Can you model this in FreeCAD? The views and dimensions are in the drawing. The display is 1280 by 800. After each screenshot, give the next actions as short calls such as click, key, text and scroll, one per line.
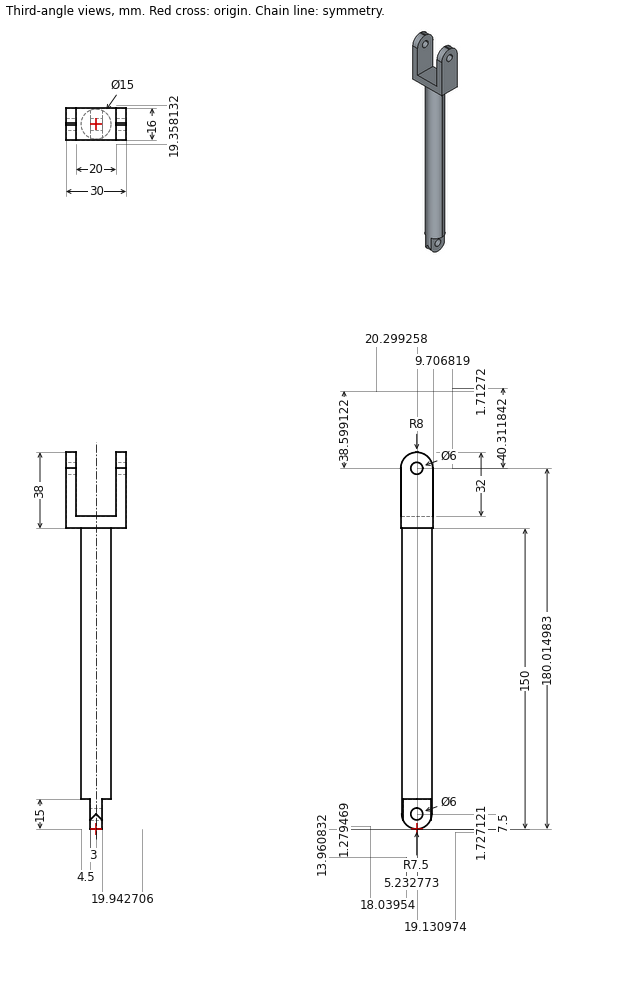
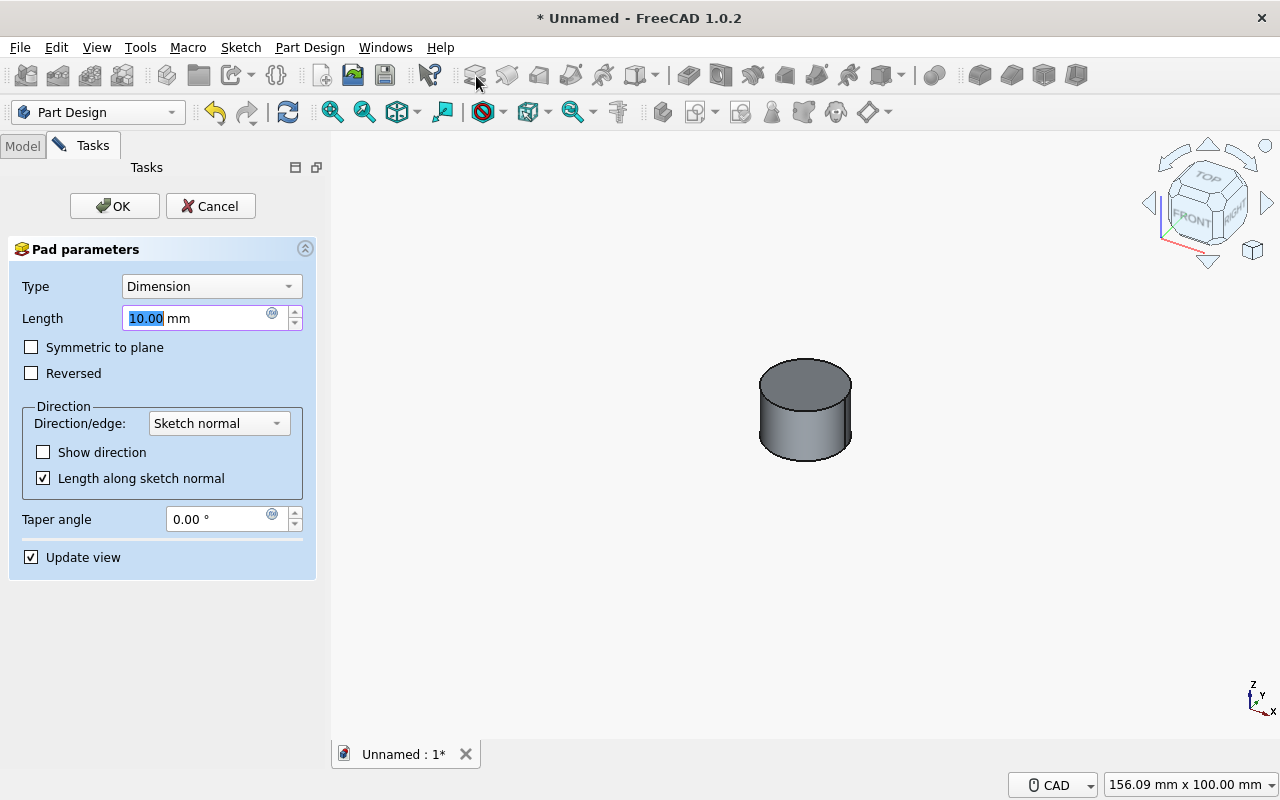
text(150)
key(Tab)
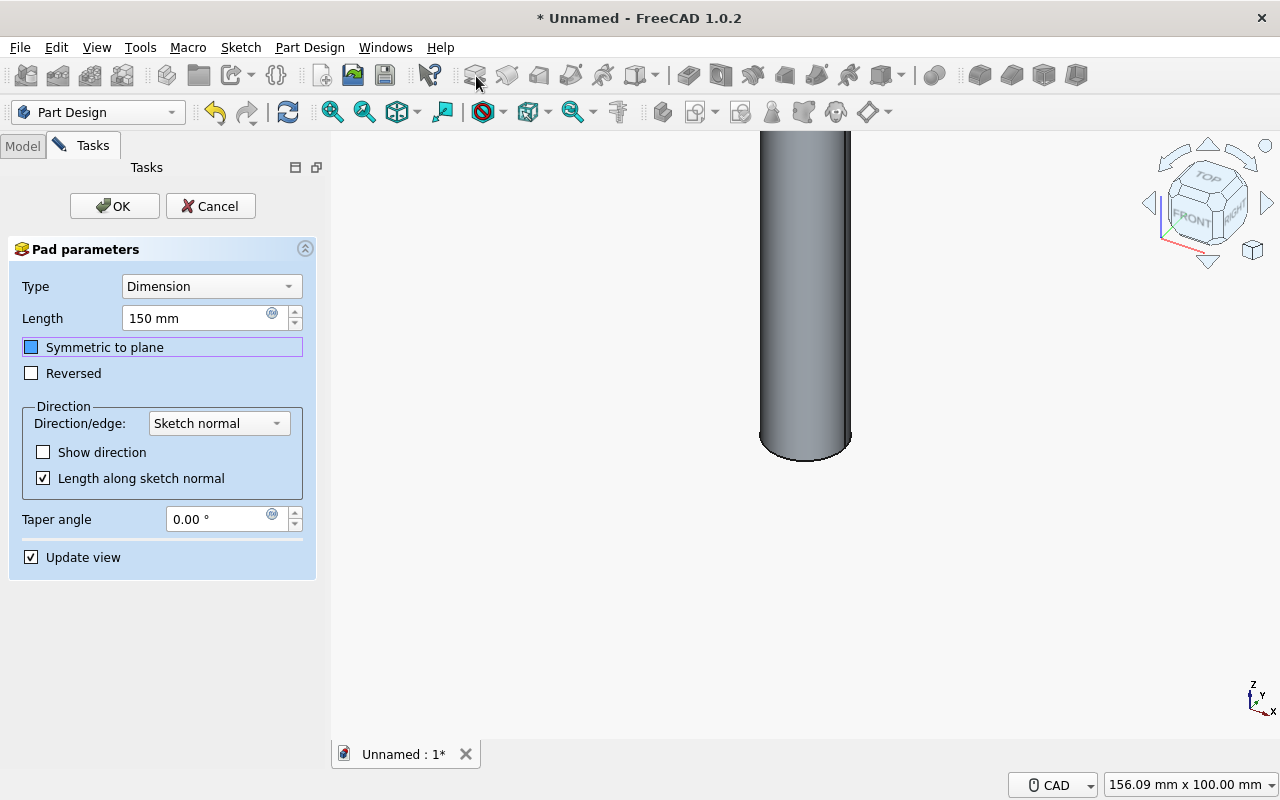
click(115, 206)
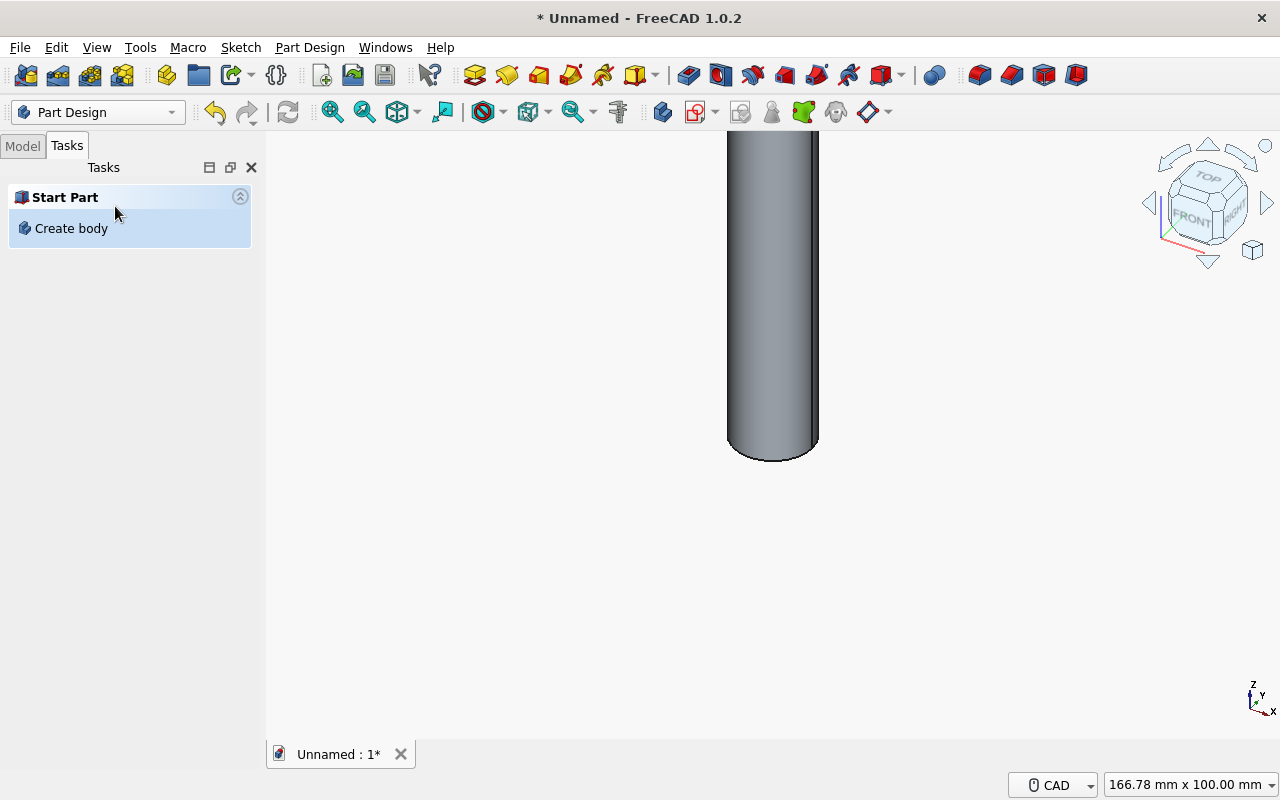
key(v)
key(f)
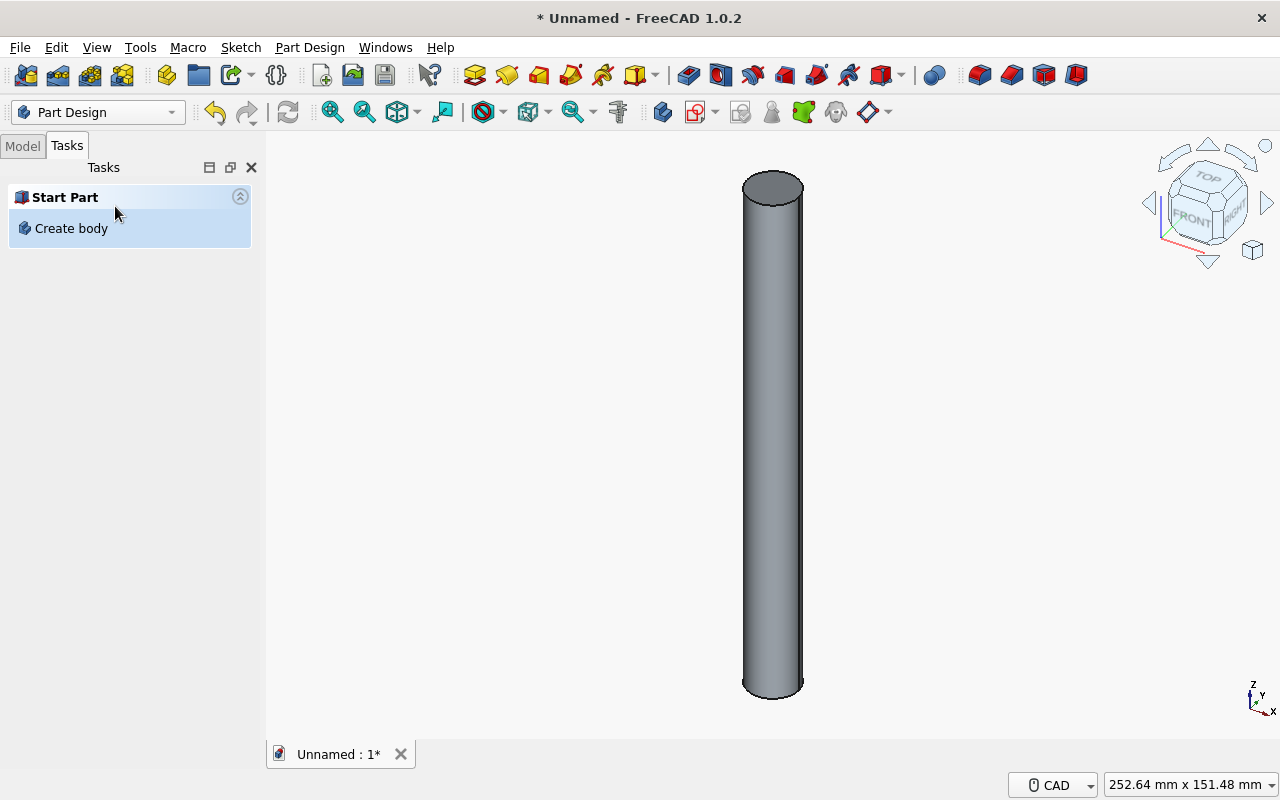
click(773, 187)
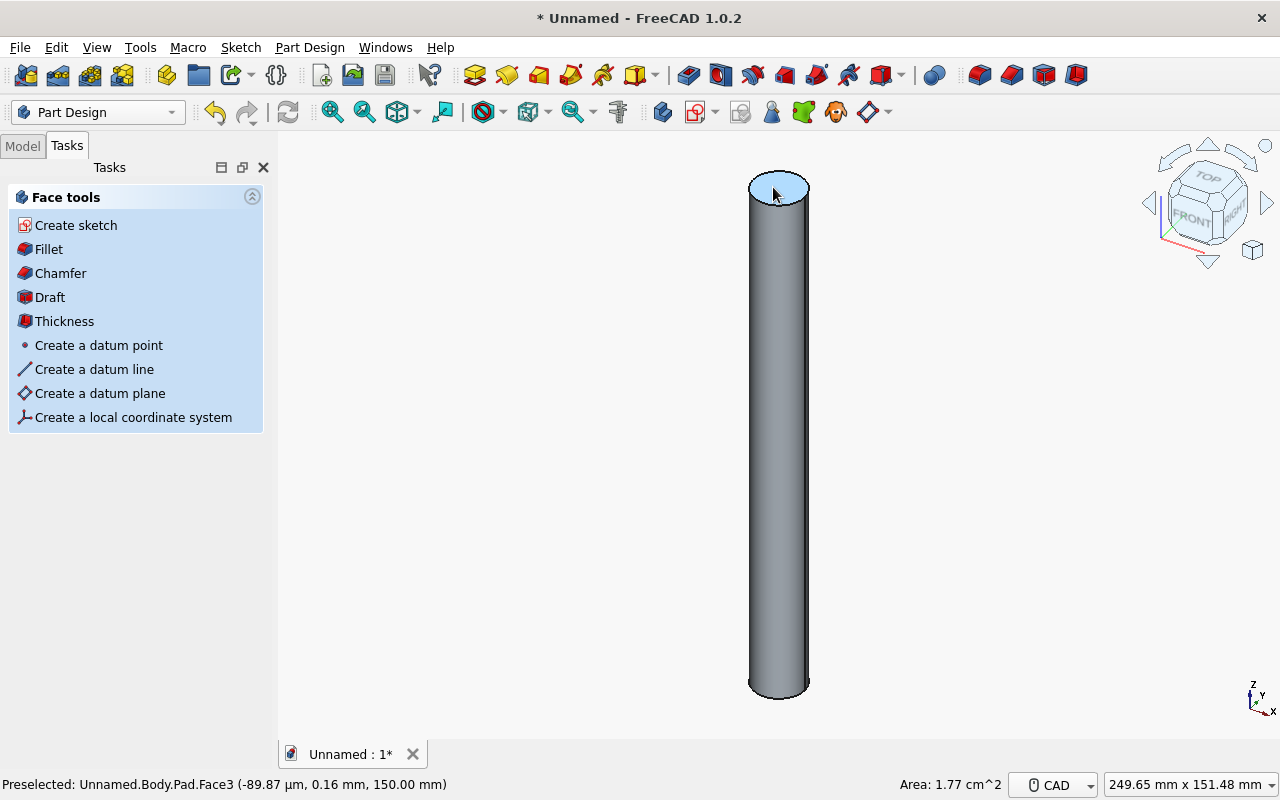
click(696, 112)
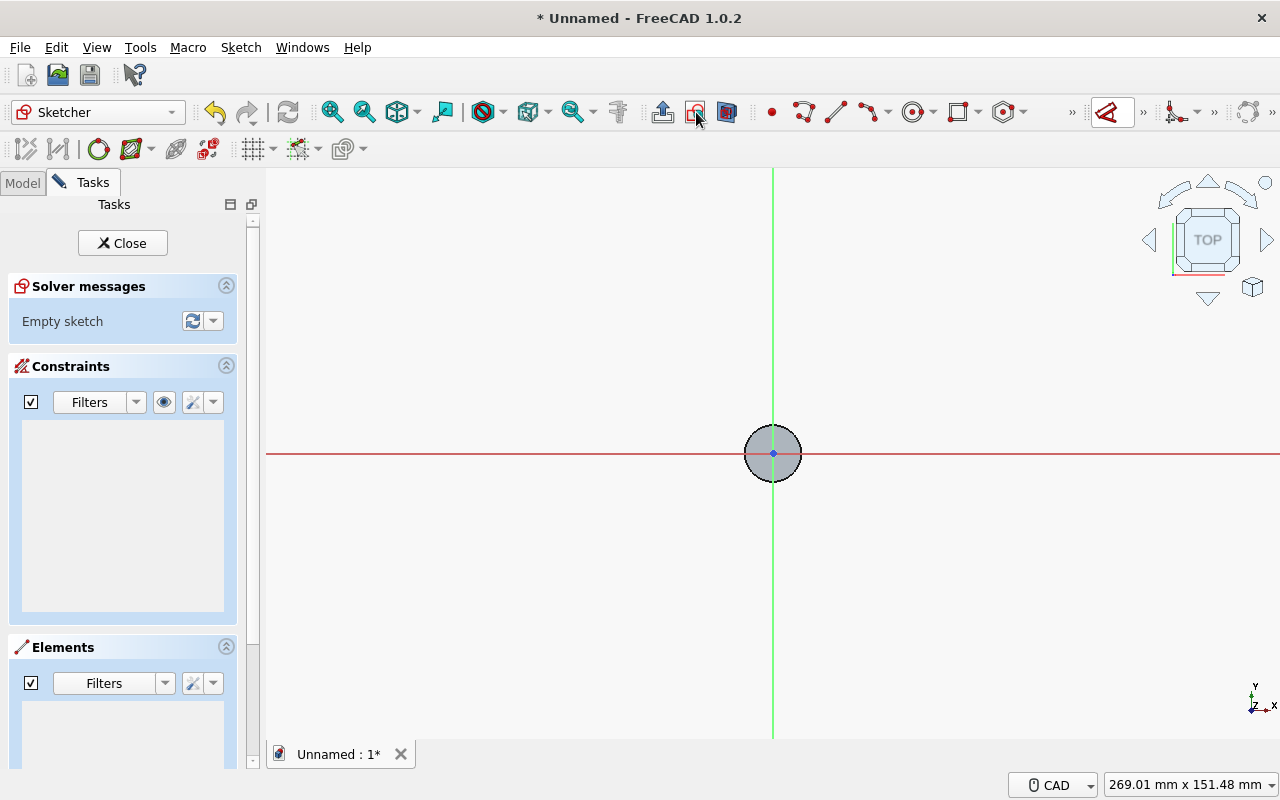
scroll(790, 453, up, 8)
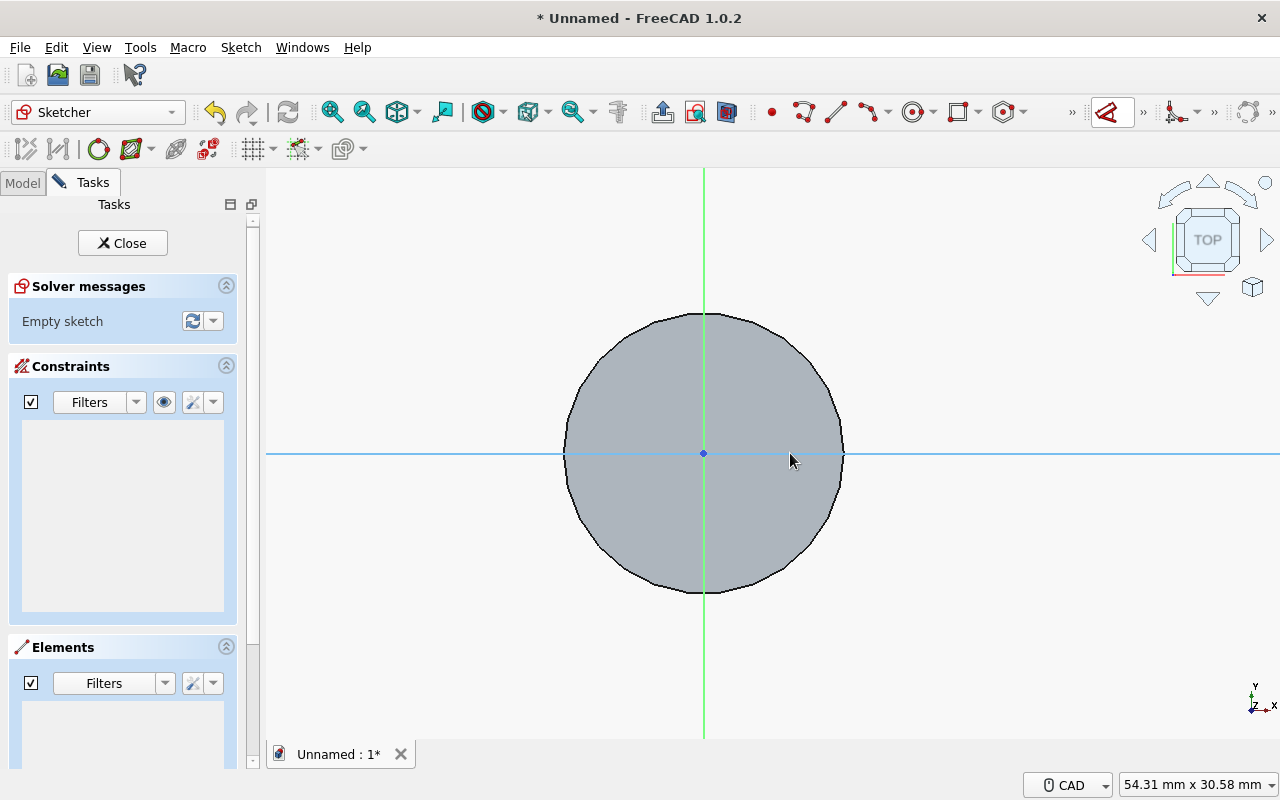
key(g)
key(v)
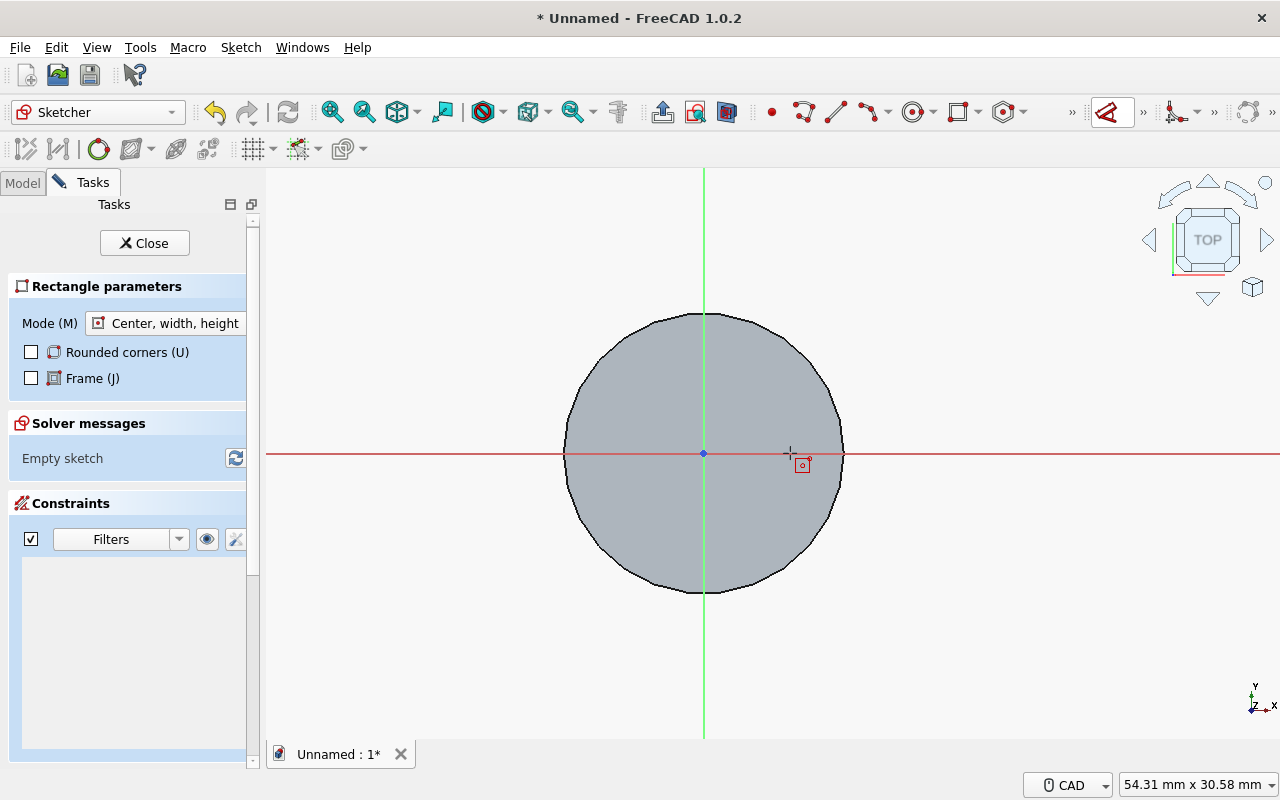
click(704, 454)
move(984, 304)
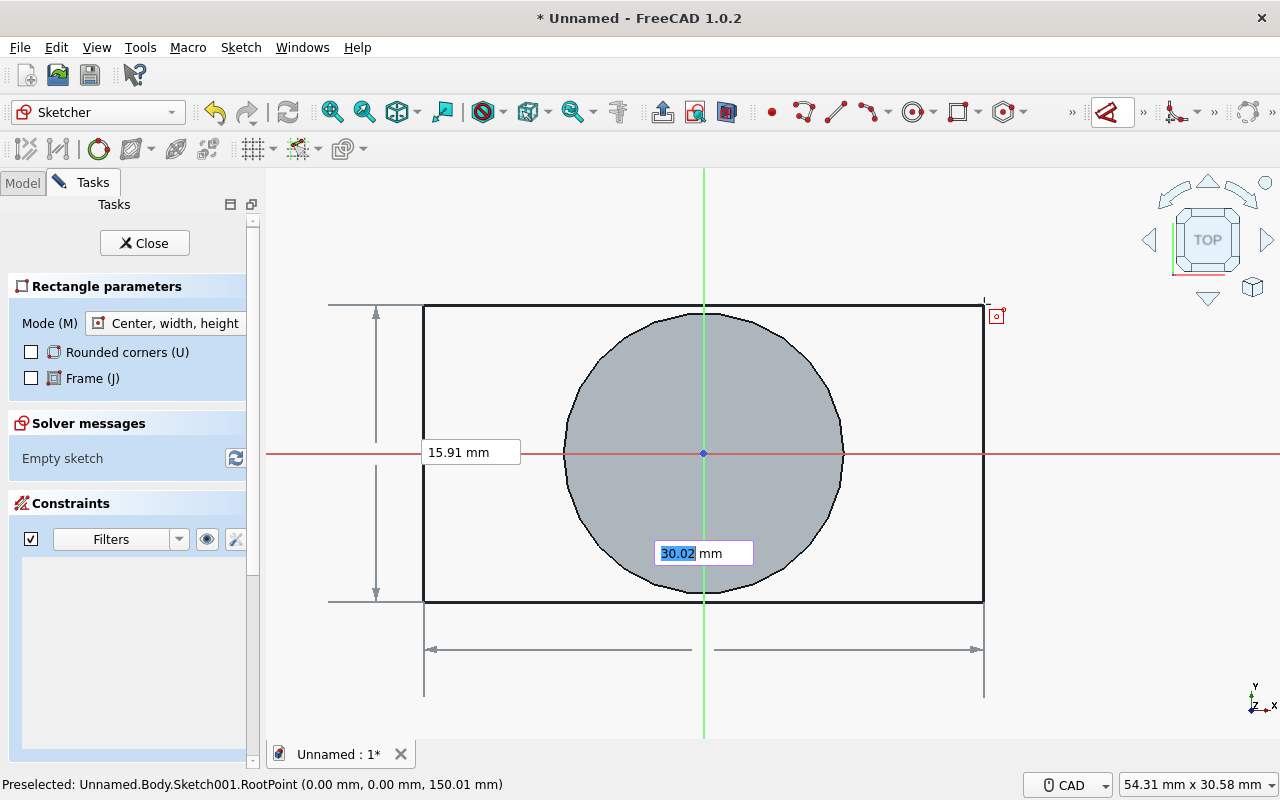
text(30)
key(Tab)
text(16)
key(Return)
key(Escape)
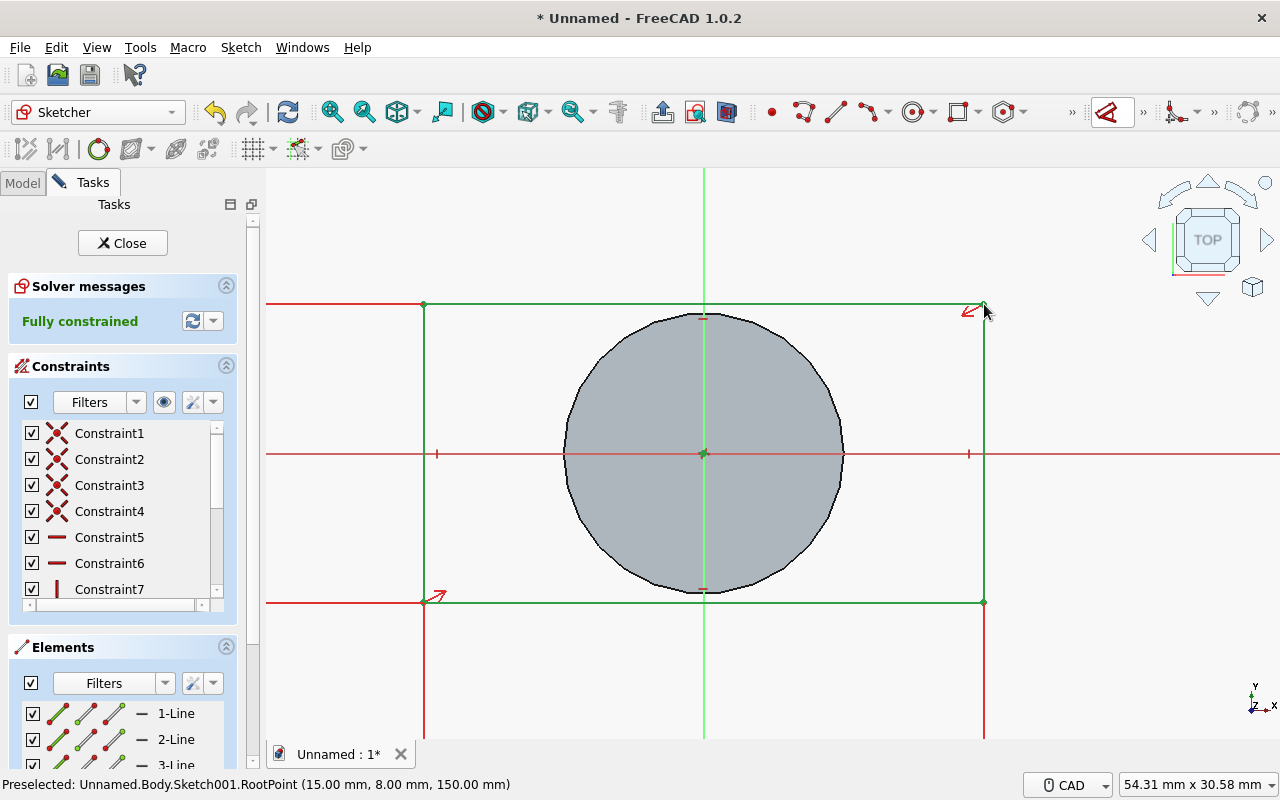
click(123, 243)